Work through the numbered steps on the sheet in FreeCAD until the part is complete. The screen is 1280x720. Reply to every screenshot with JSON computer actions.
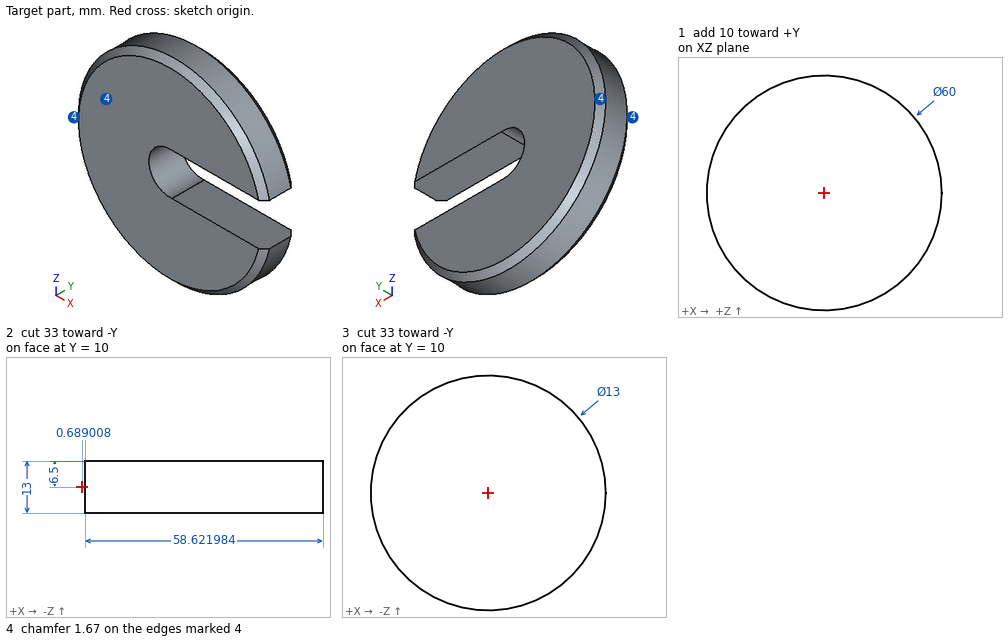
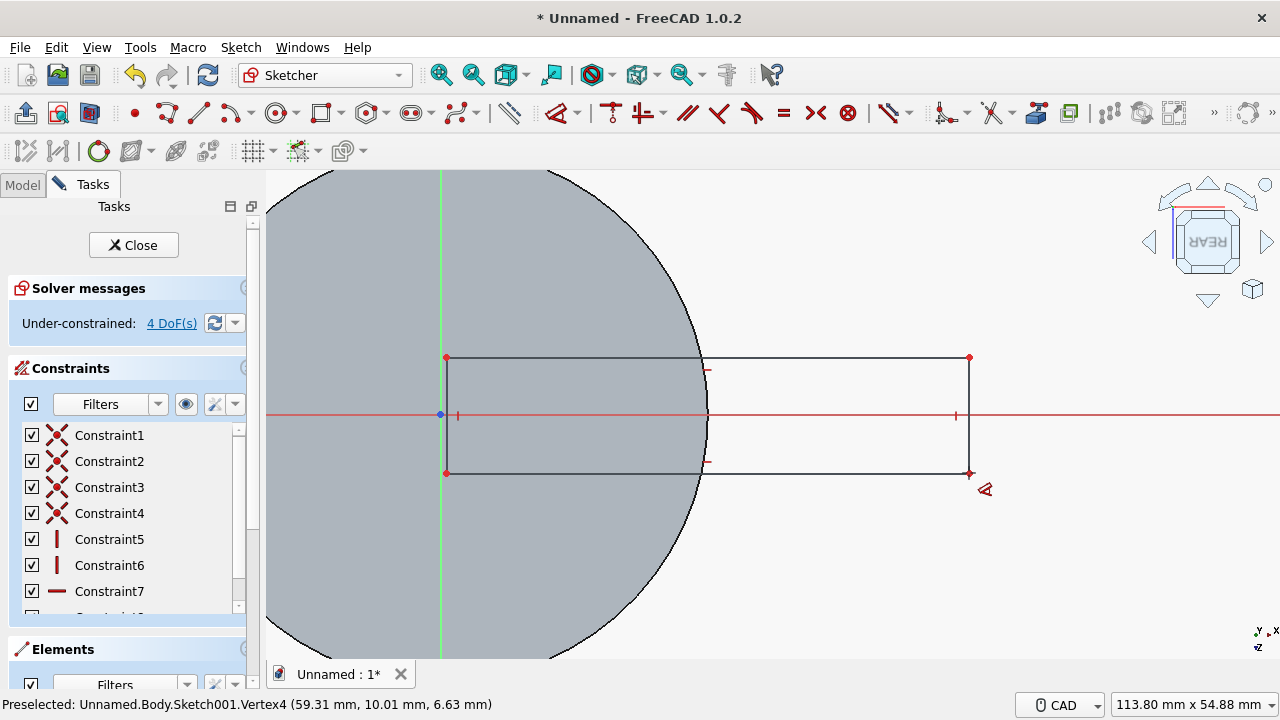
{"action": "scroll", "coordinate": [447, 392], "scroll_direction": "up", "scroll_amount": 5}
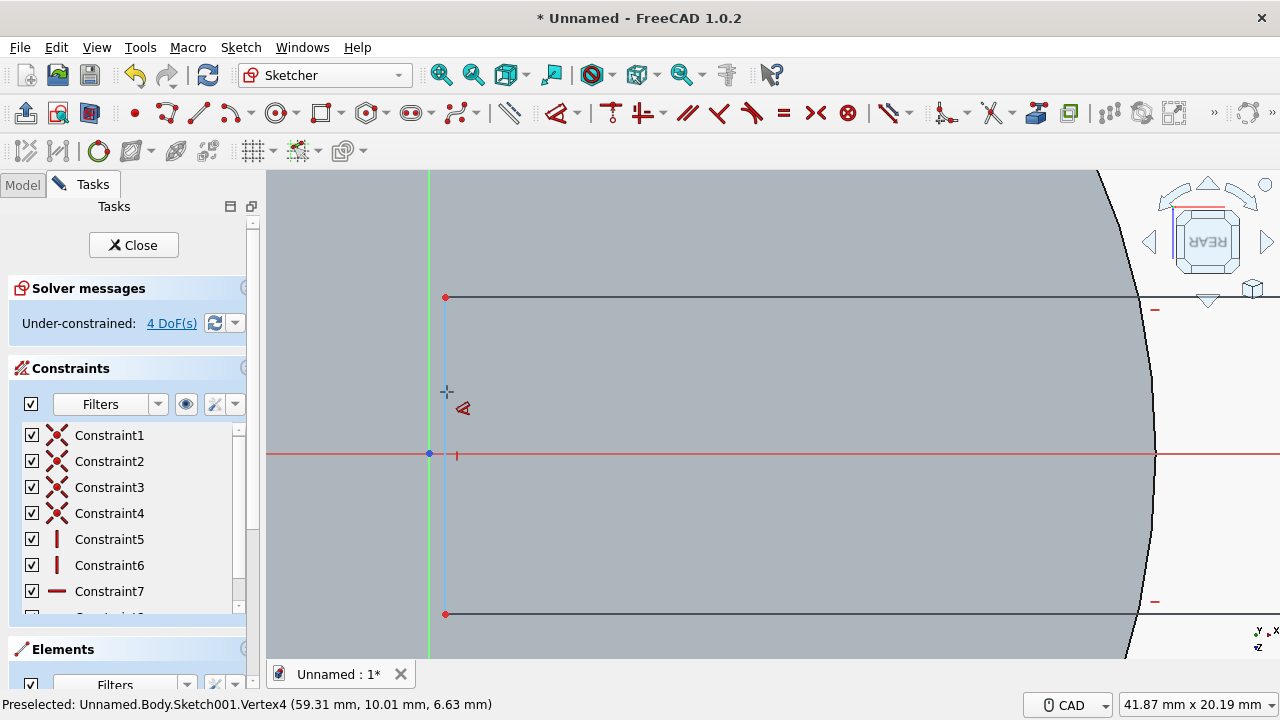
{"action": "left_click", "coordinate": [445, 392]}
{"action": "left_click", "coordinate": [411, 383]}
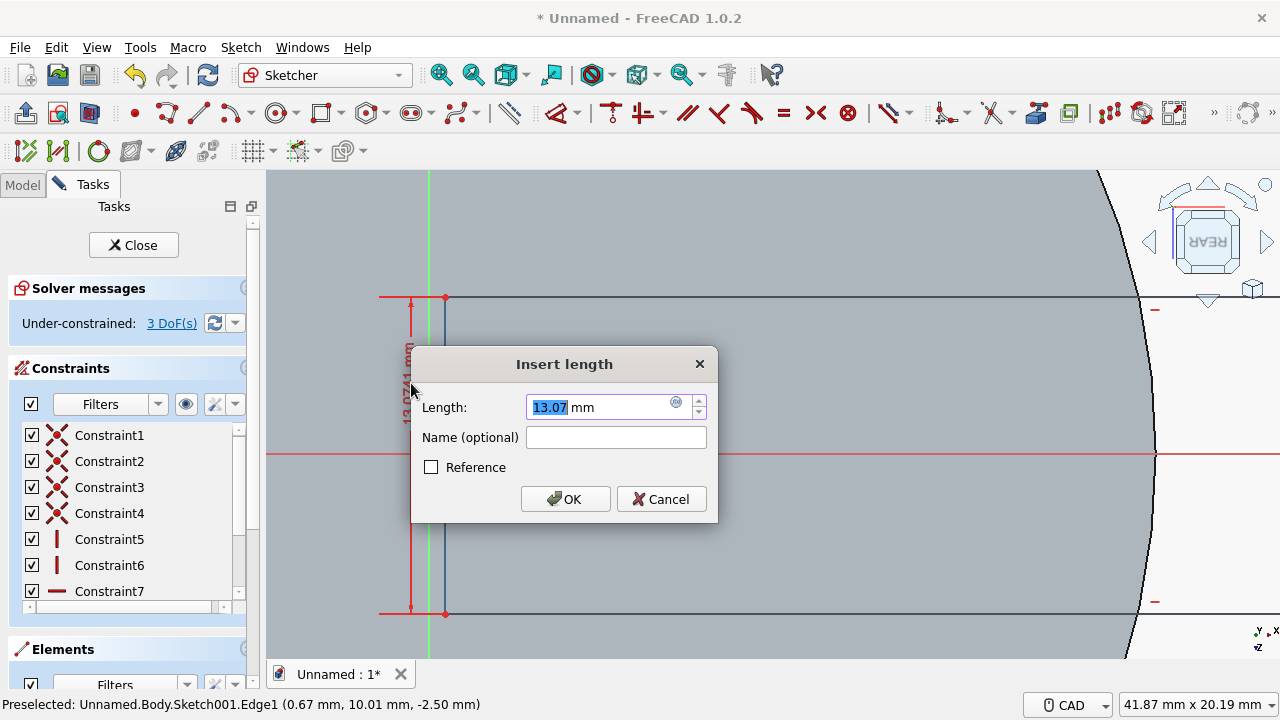
{"action": "type", "text": "13"}
{"action": "key", "text": "Return"}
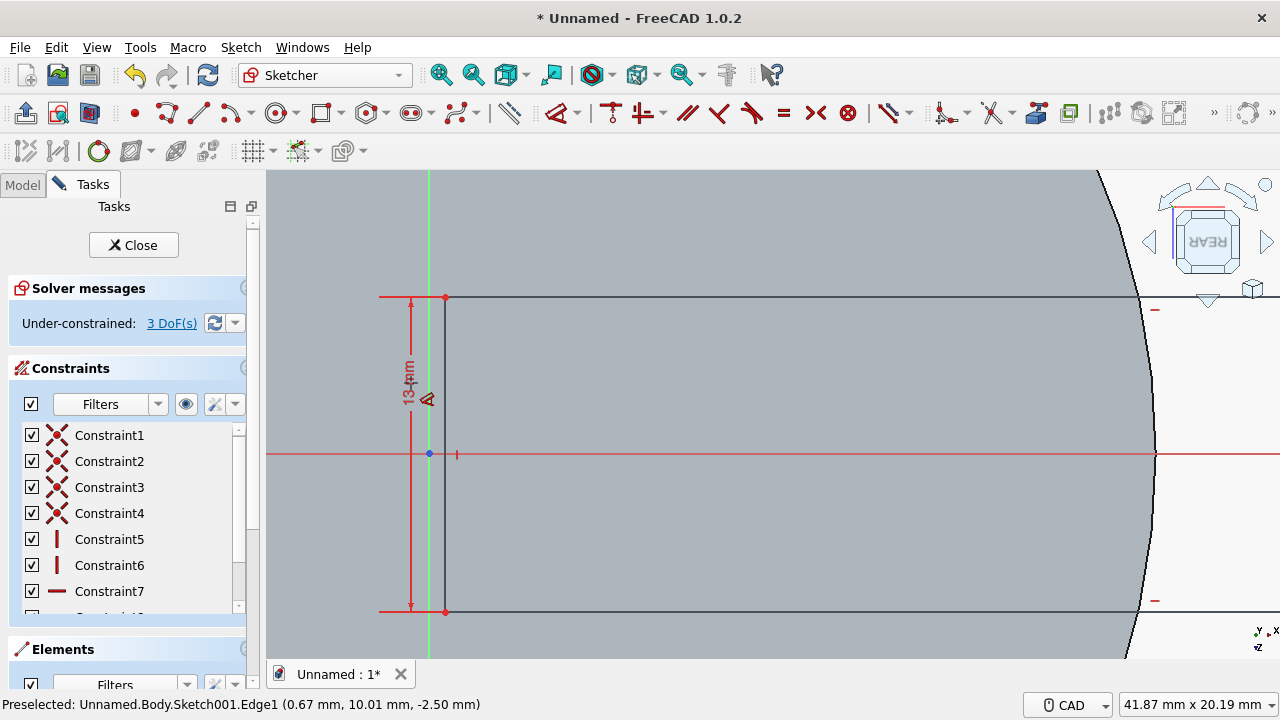
{"action": "left_click", "coordinate": [445, 297]}
{"action": "left_click", "coordinate": [395, 340]}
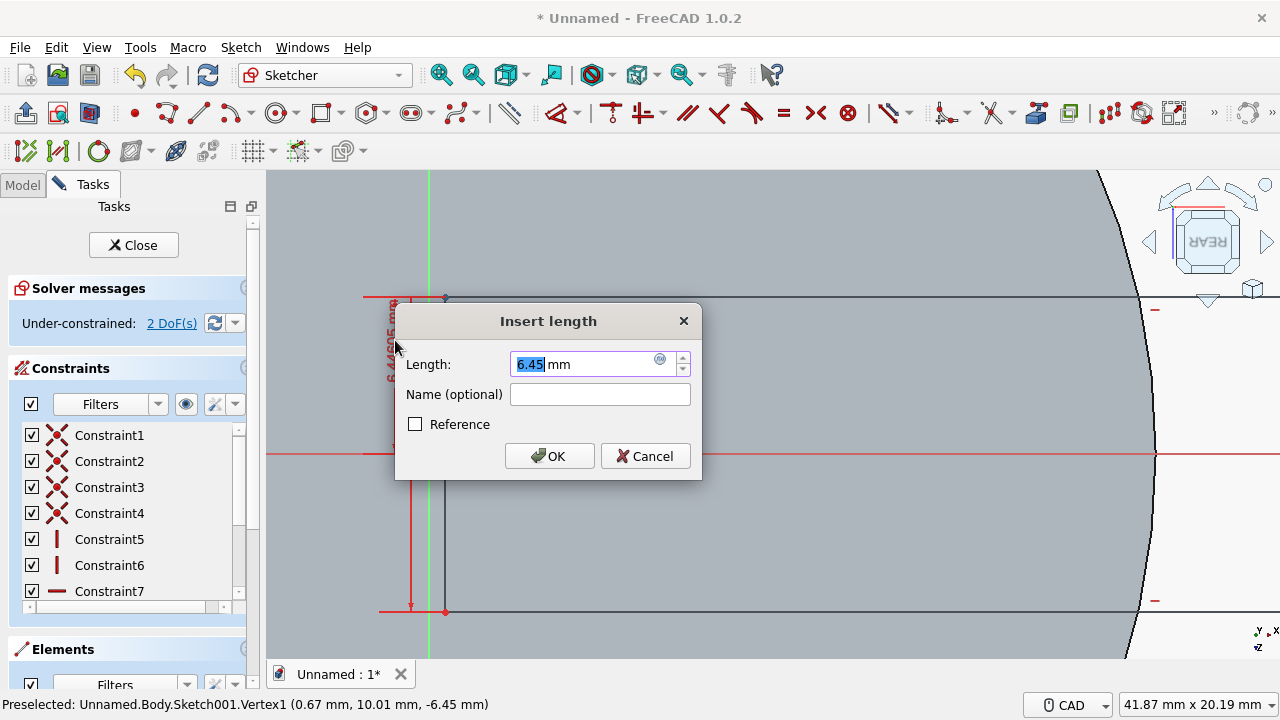
{"action": "type", "text": "6.5"}
{"action": "key", "text": "Return"}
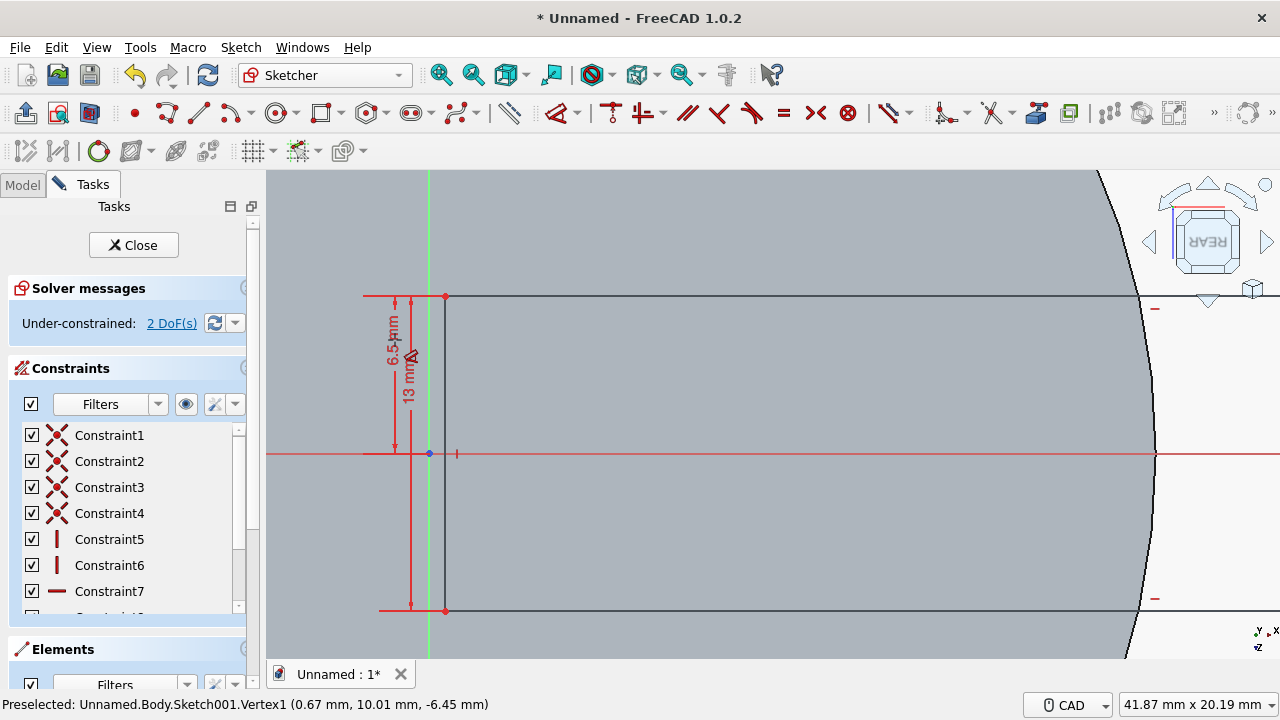
{"action": "left_click", "coordinate": [871, 611]}
{"action": "left_click", "coordinate": [780, 577]}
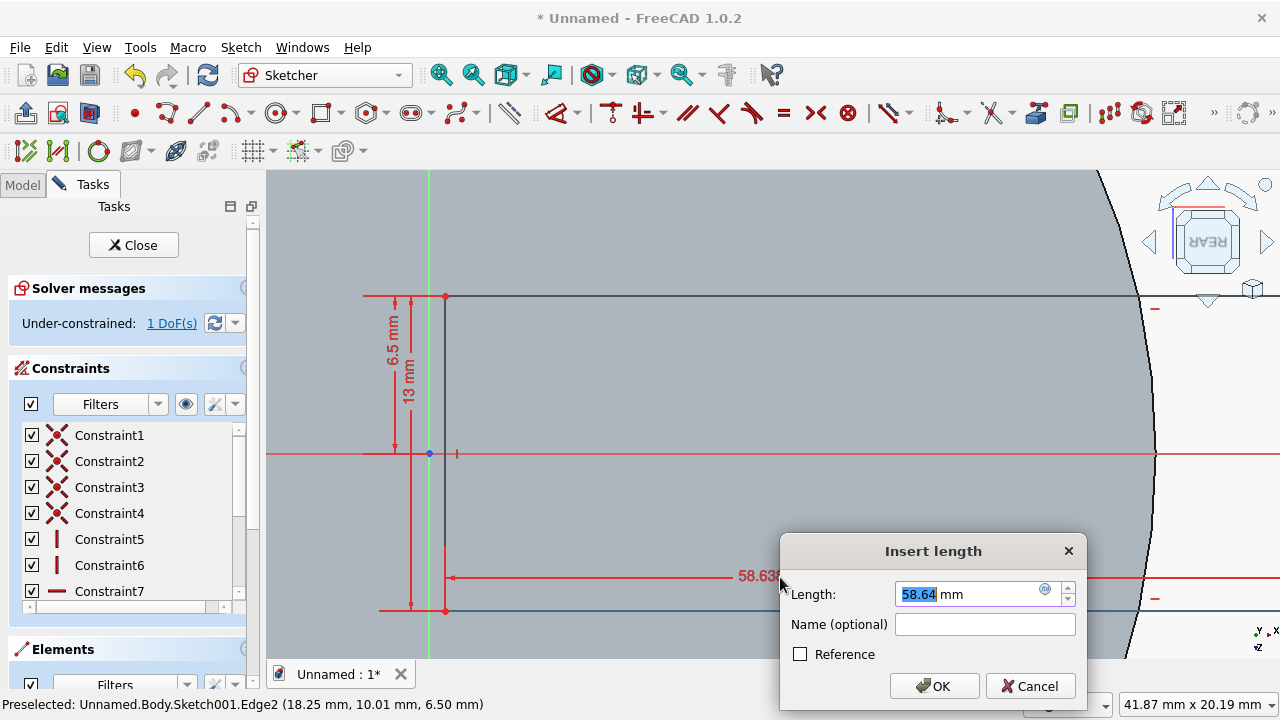
{"action": "type", "text": "58.621984"}
{"action": "key", "text": "Return"}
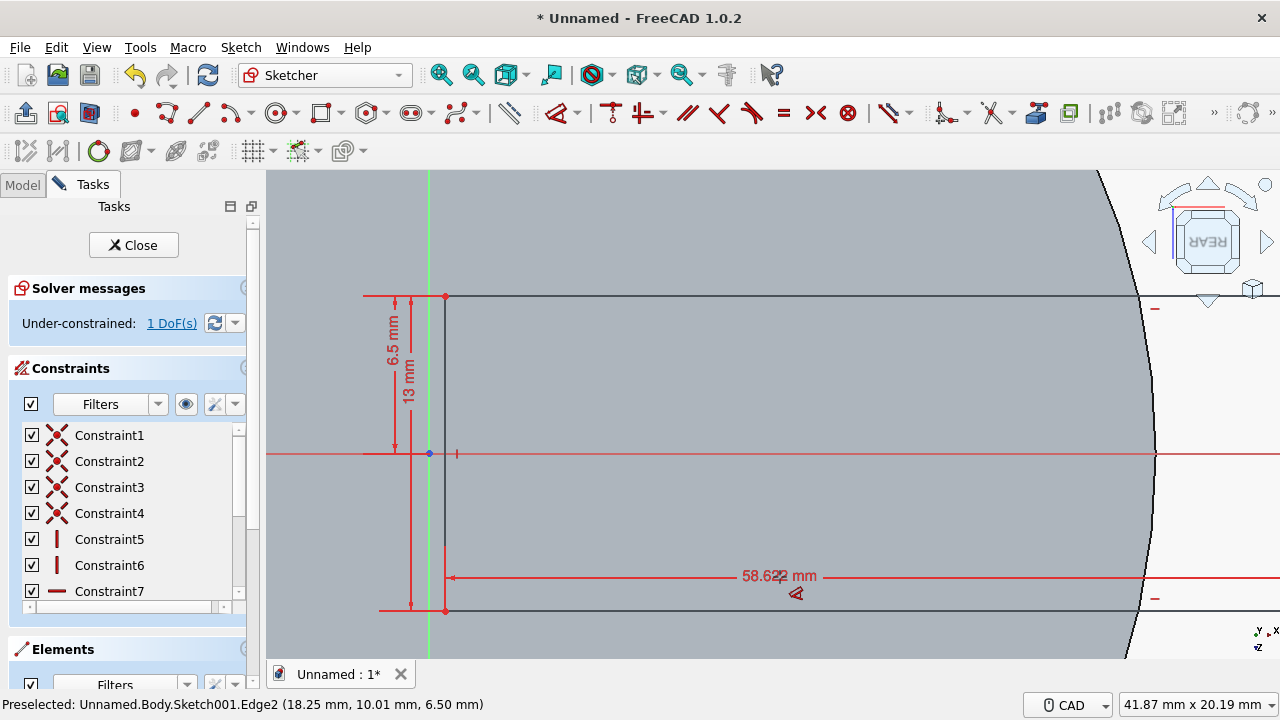
{"action": "scroll", "coordinate": [445, 296], "scroll_direction": "up", "scroll_amount": 5}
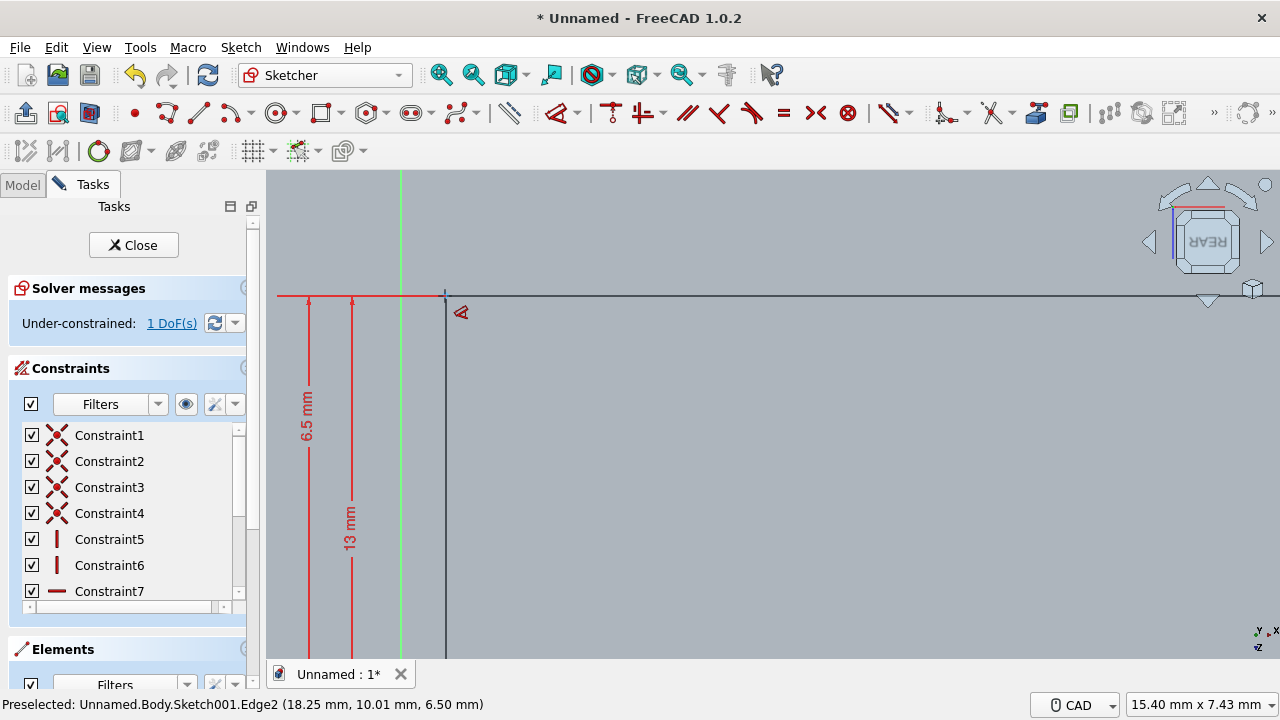
{"action": "left_click", "coordinate": [446, 296]}
{"action": "left_click", "coordinate": [424, 262]}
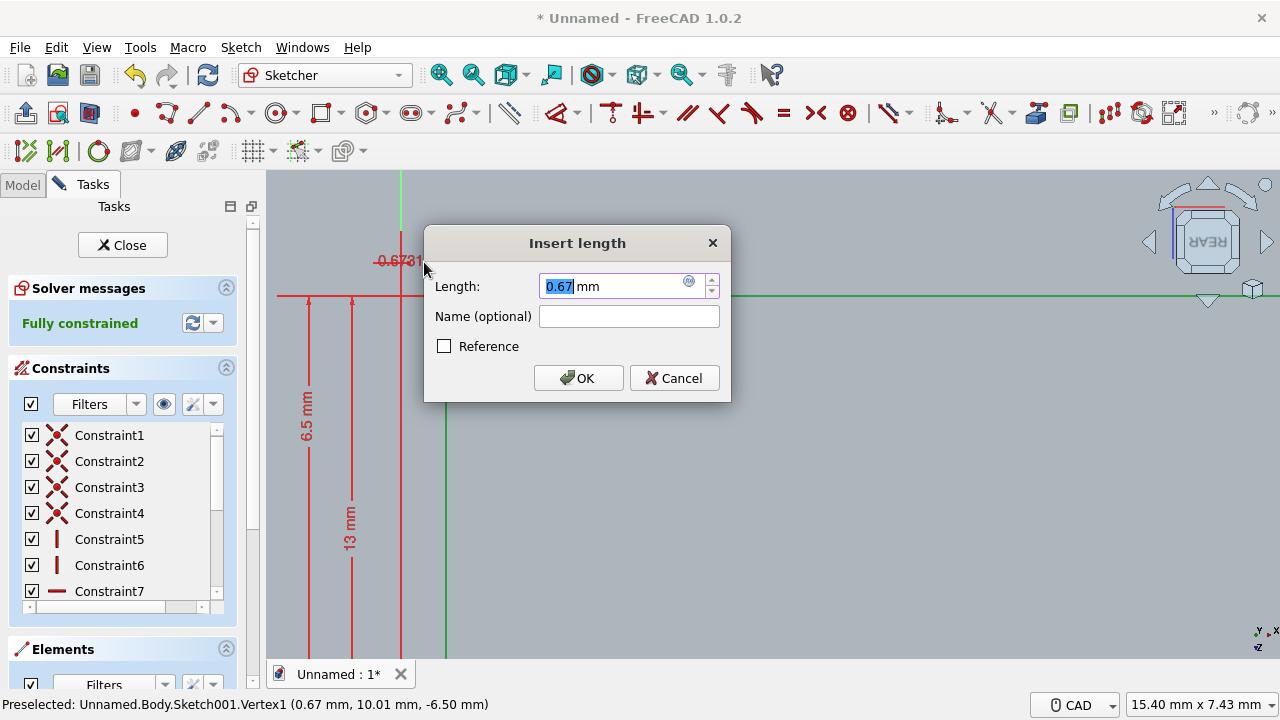
{"action": "type", "text": "0.689008"}
{"action": "key", "text": "Return"}
{"action": "key", "text": "Escape"}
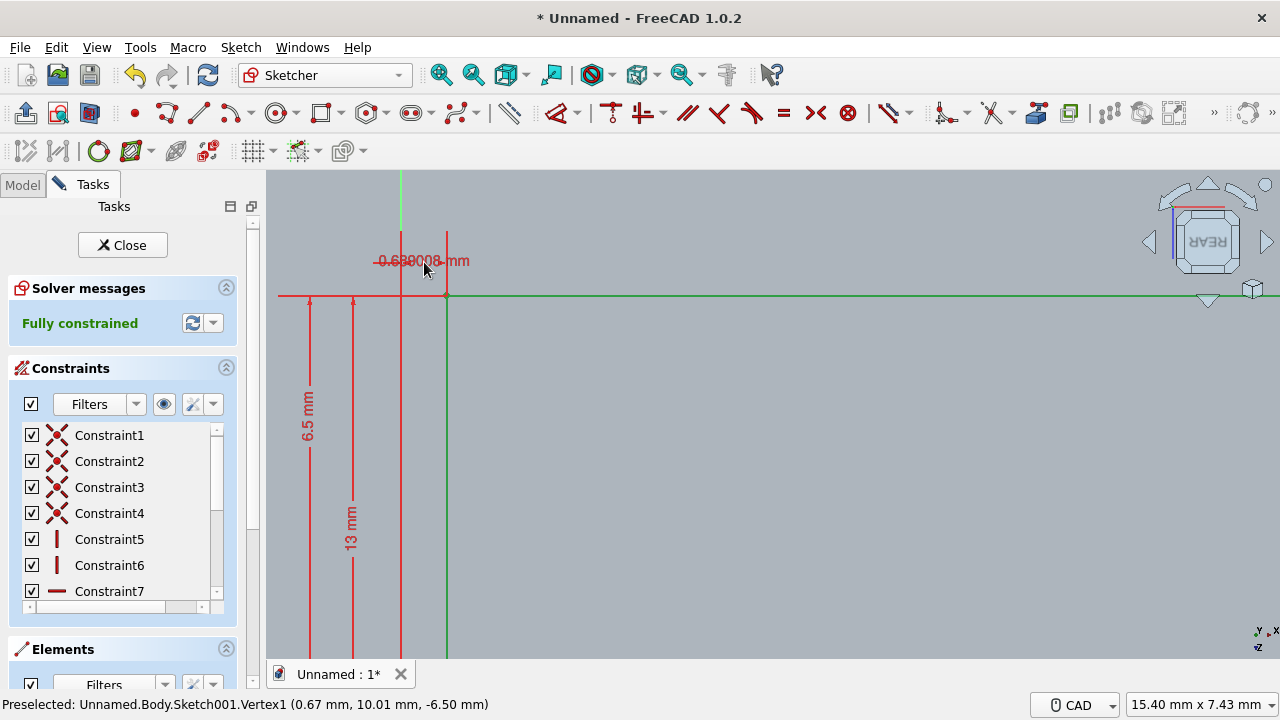
{"action": "left_click", "coordinate": [123, 245]}